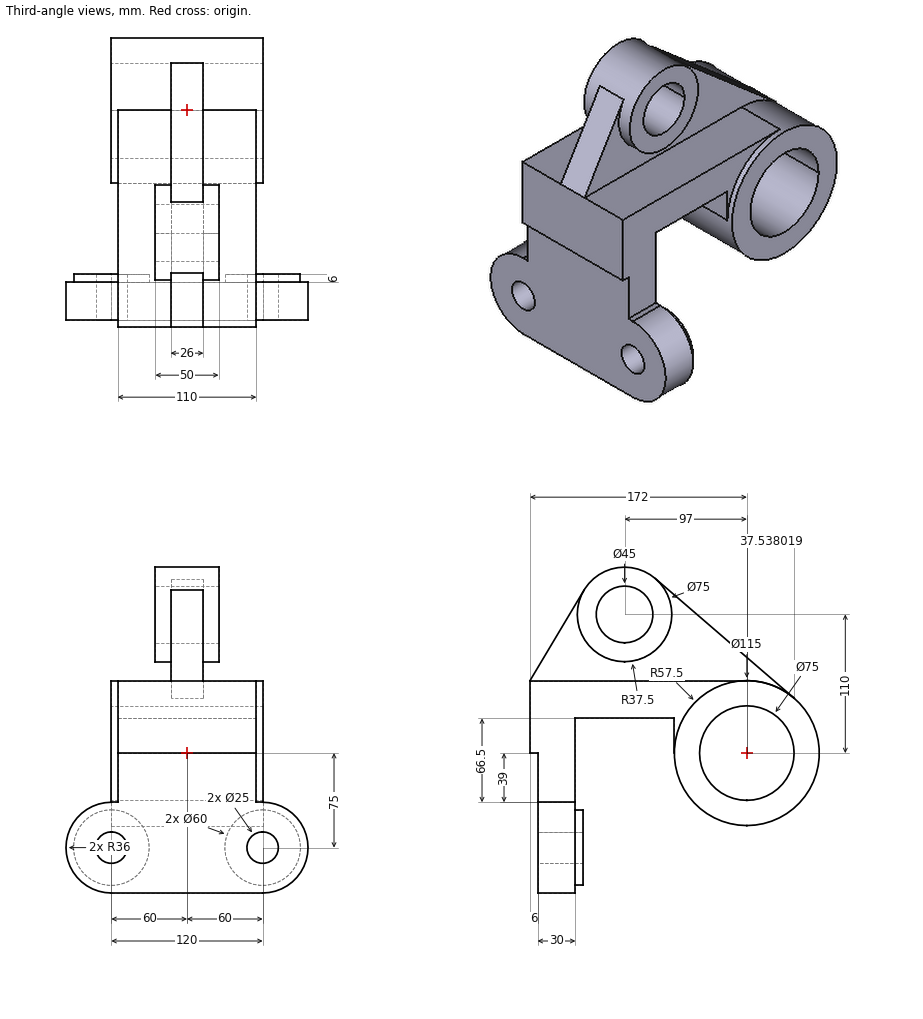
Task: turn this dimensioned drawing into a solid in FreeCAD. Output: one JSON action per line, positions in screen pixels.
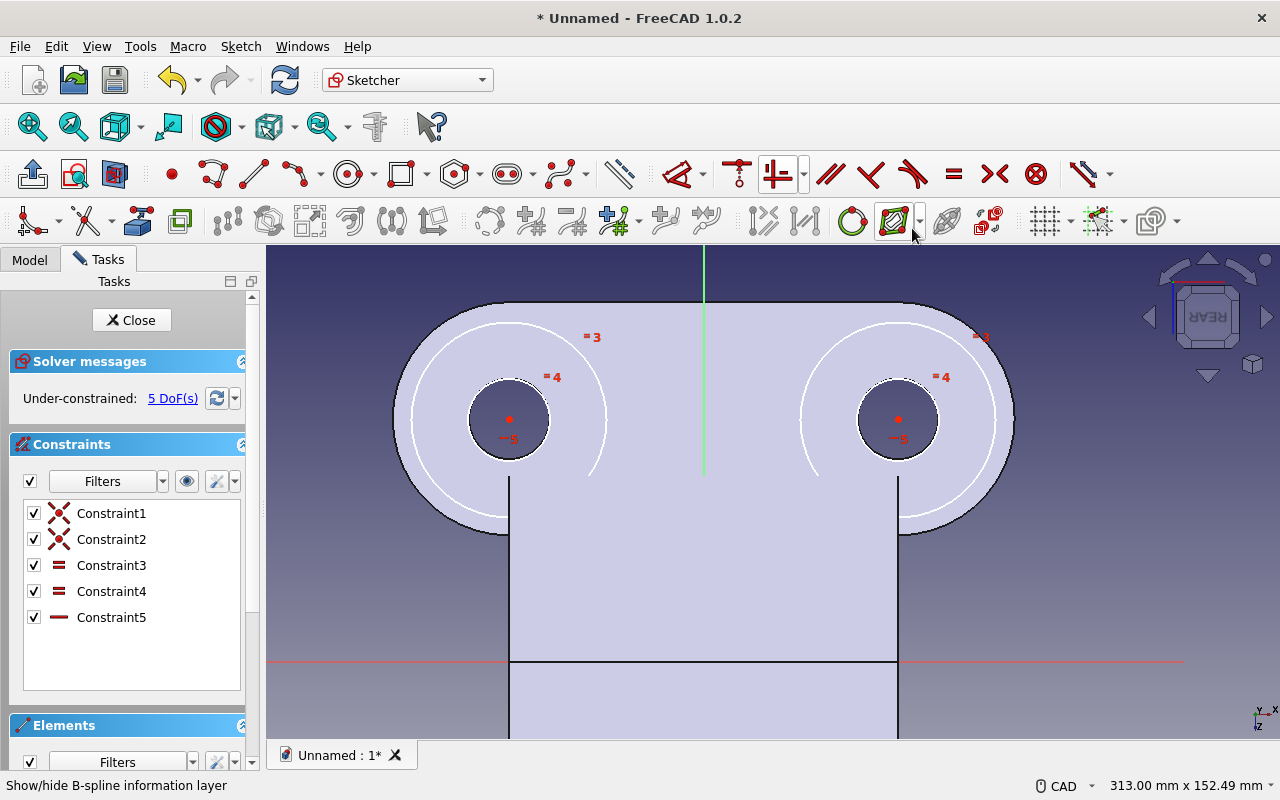
{"action": "left_click", "coordinate": [676, 174]}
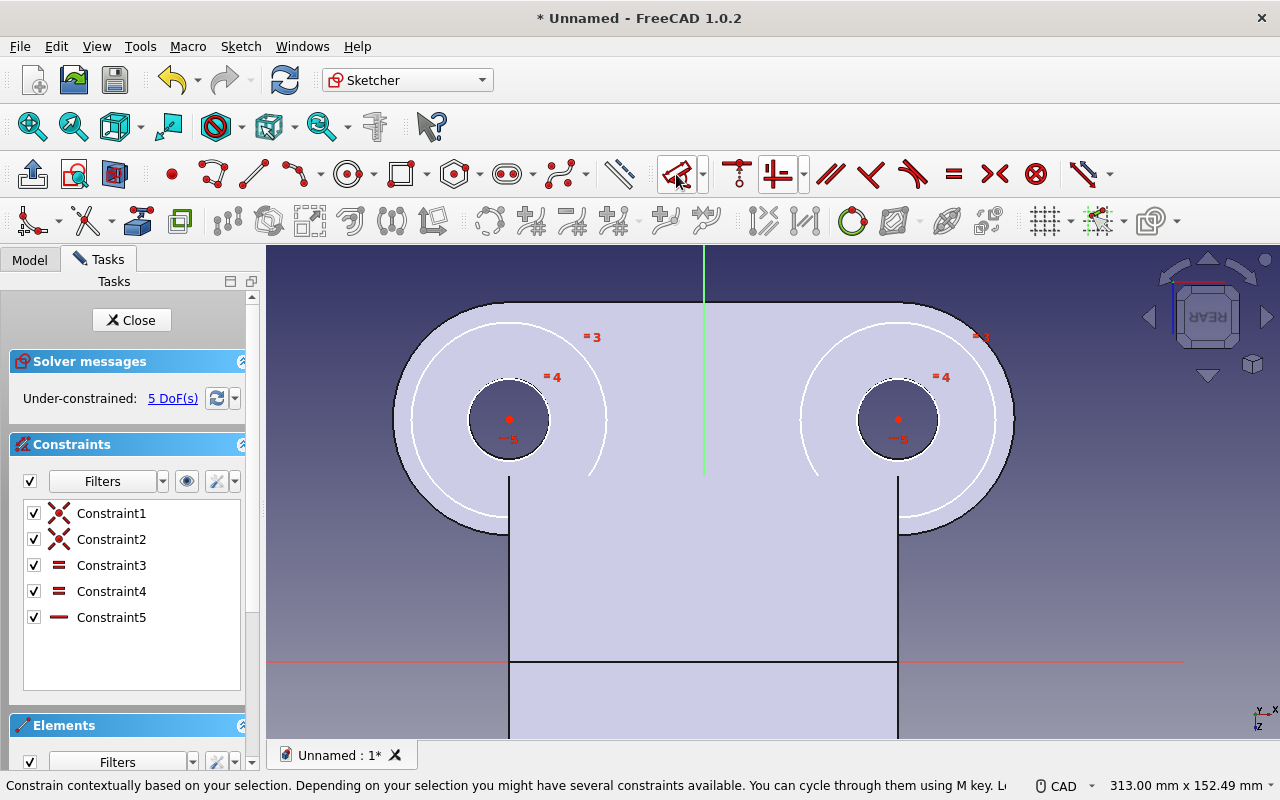
{"action": "left_click", "coordinate": [967, 351]}
{"action": "left_click", "coordinate": [990, 328]}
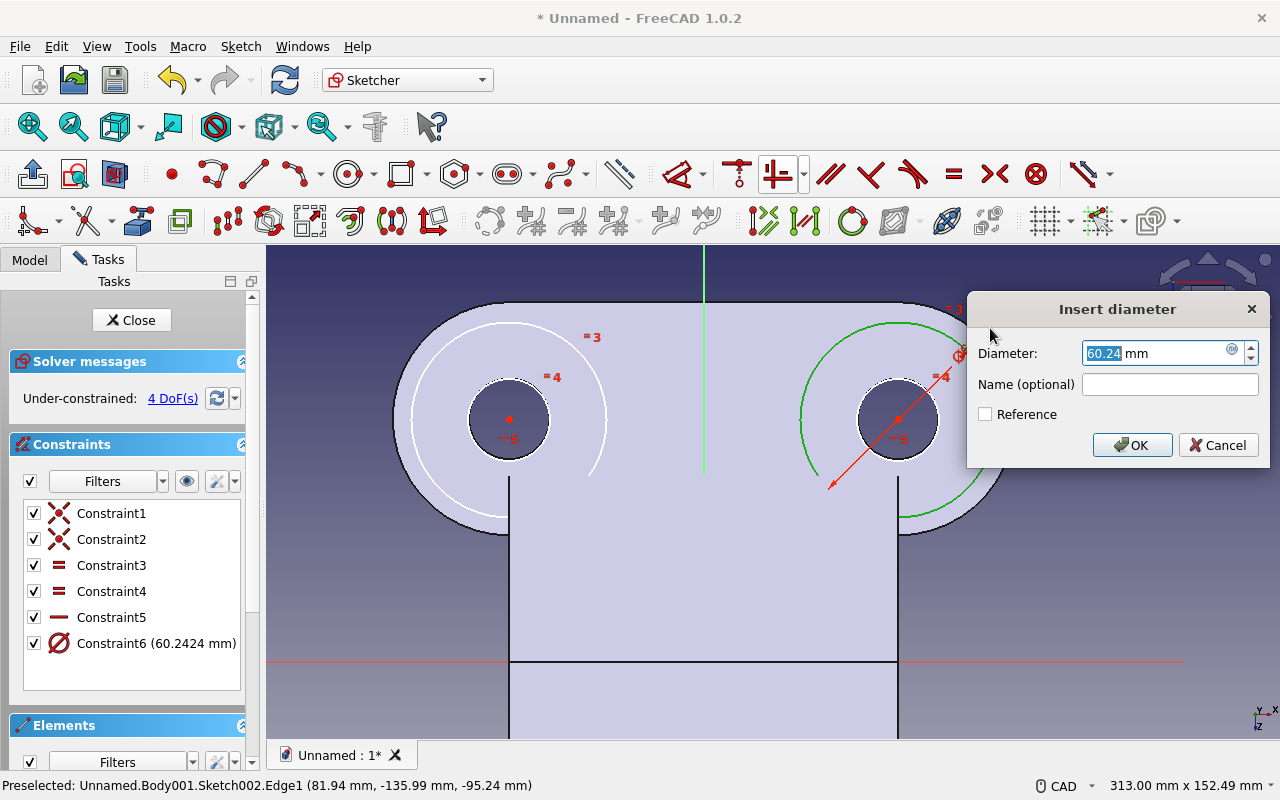
{"action": "type", "text": "60"}
{"action": "key", "text": "Return"}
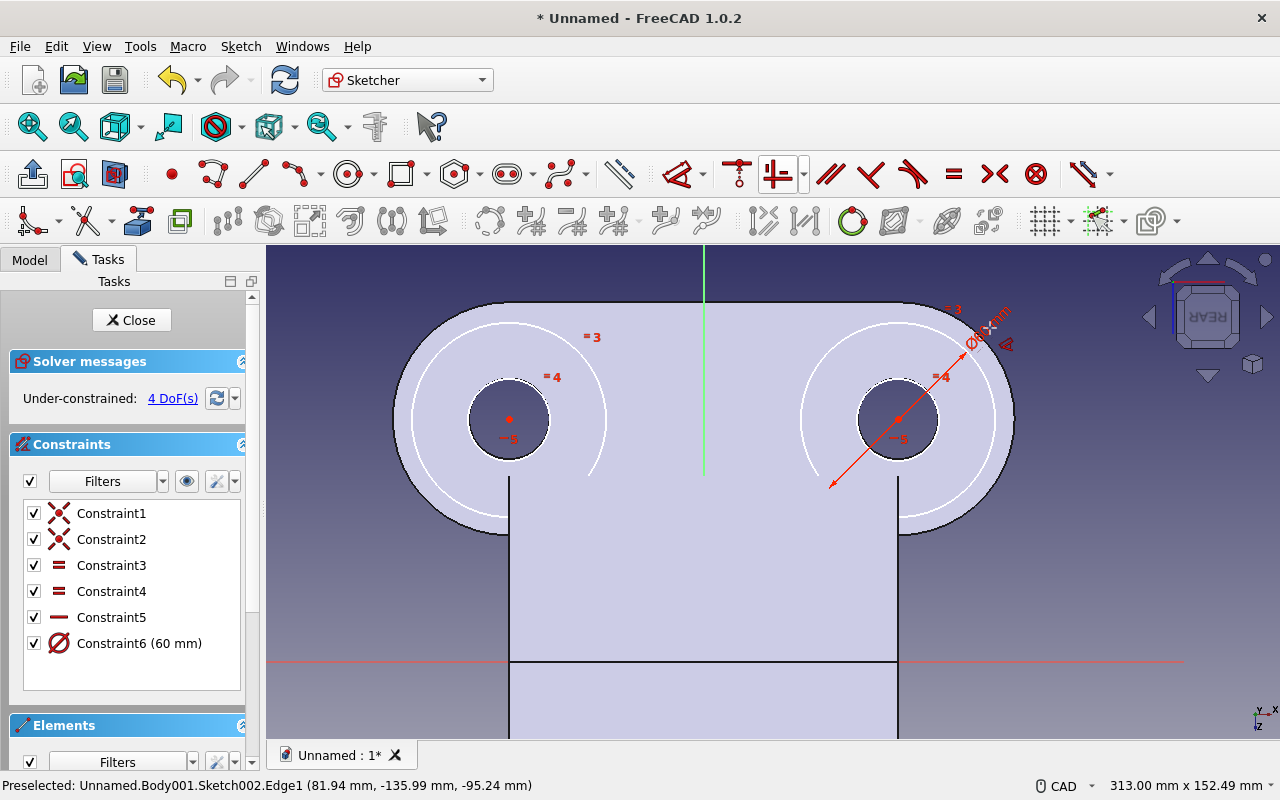
{"action": "left_click", "coordinate": [927, 391]}
{"action": "left_click", "coordinate": [950, 368]}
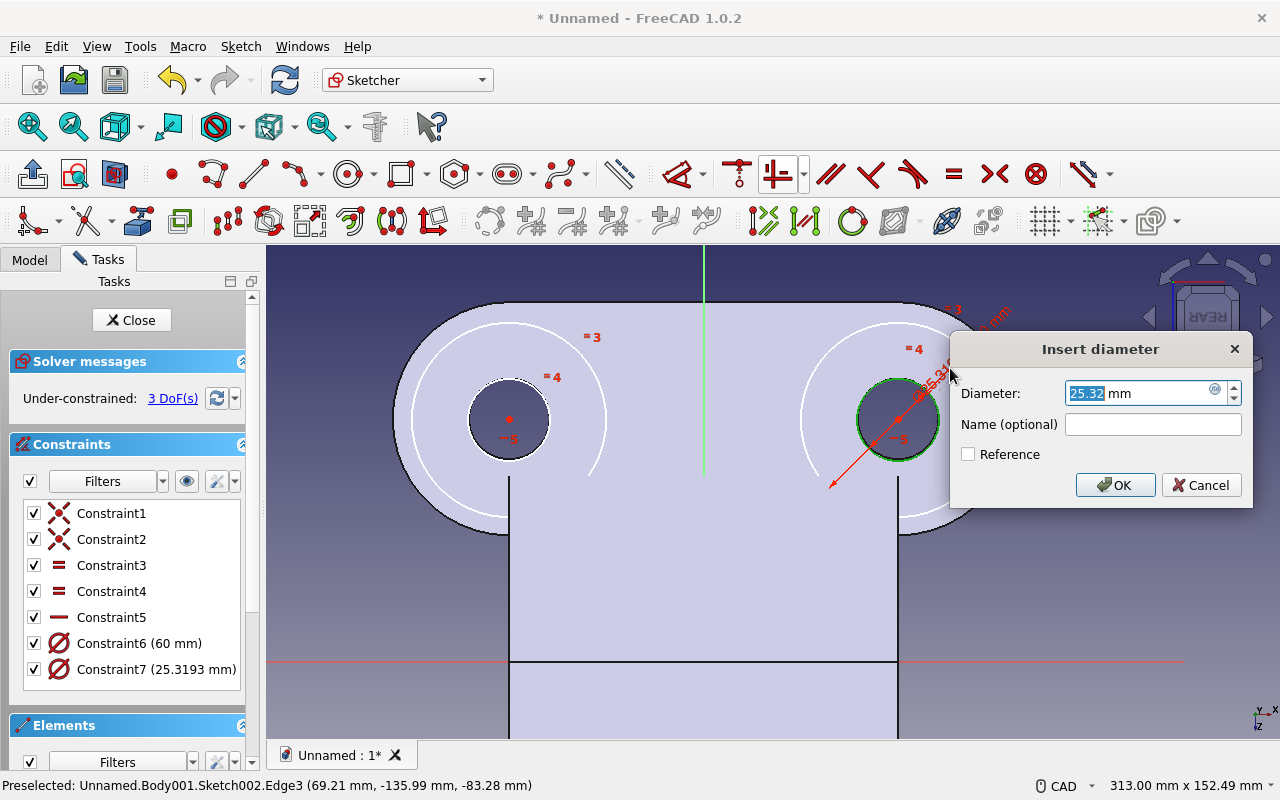
{"action": "type", "text": "25"}
{"action": "key", "text": "Return"}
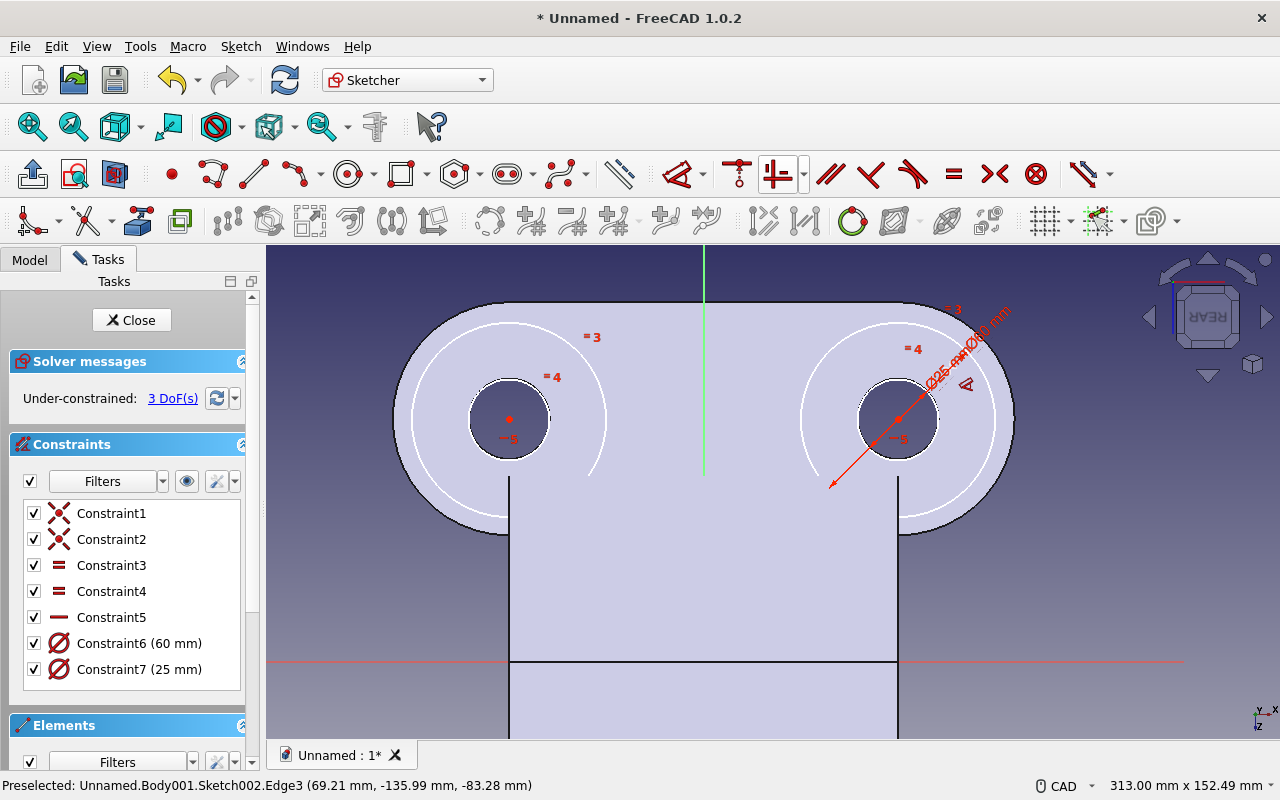
{"action": "left_click", "coordinate": [898, 420]}
{"action": "left_click", "coordinate": [801, 696]}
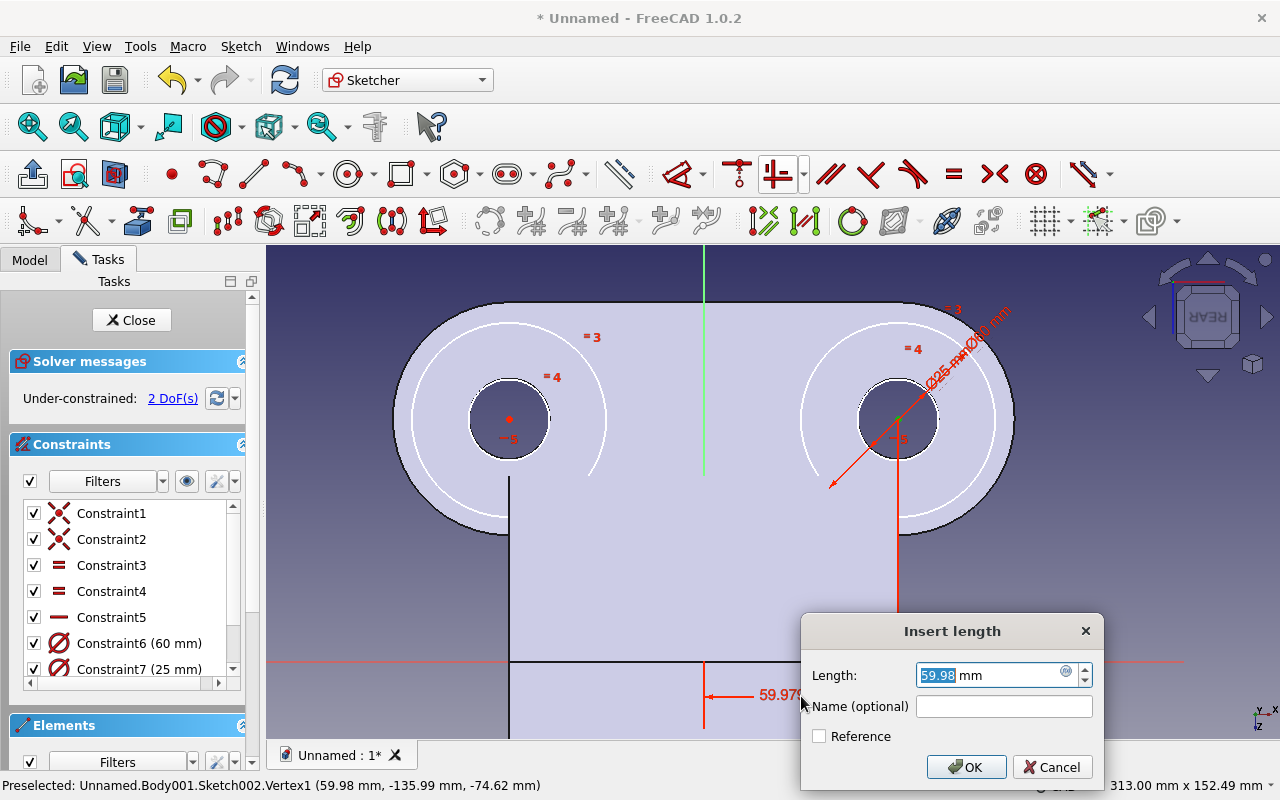
{"action": "type", "text": "60"}
{"action": "key", "text": "Return"}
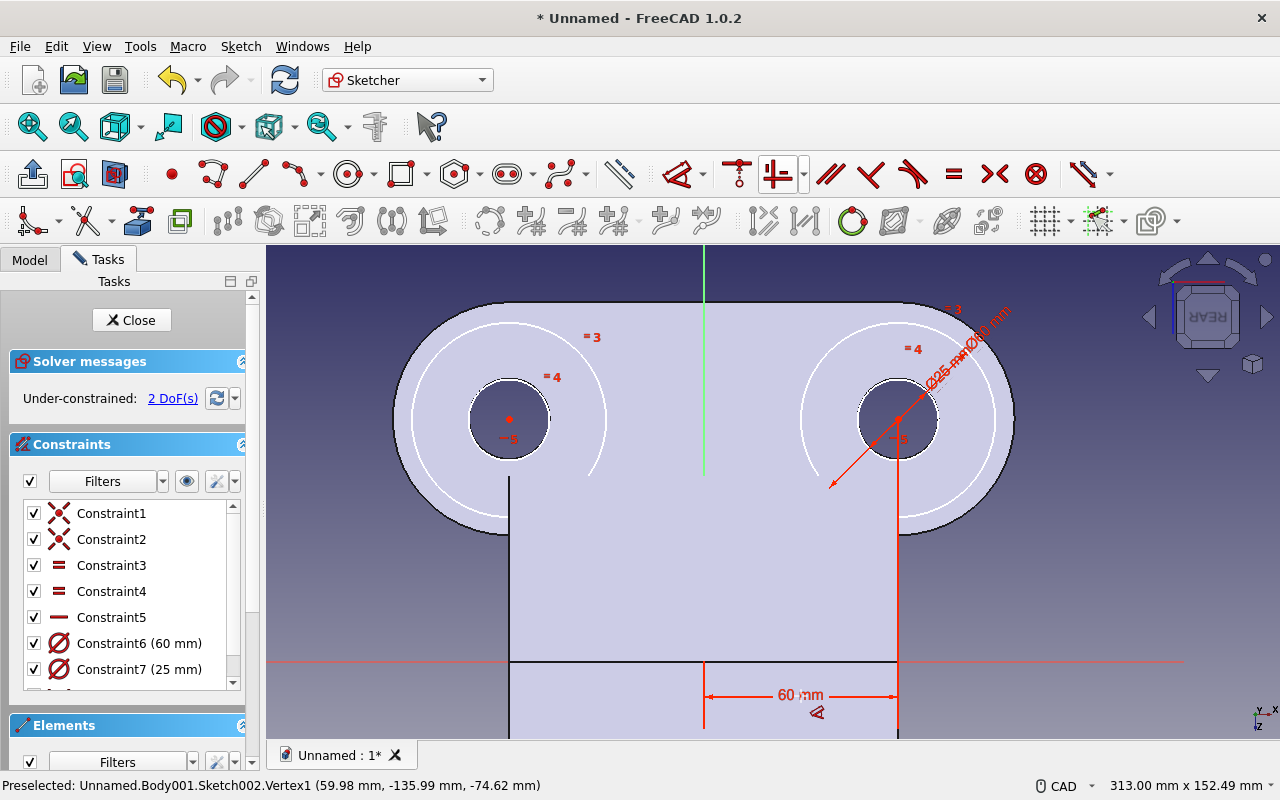
{"action": "left_click", "coordinate": [898, 420]}
{"action": "left_click", "coordinate": [932, 541]}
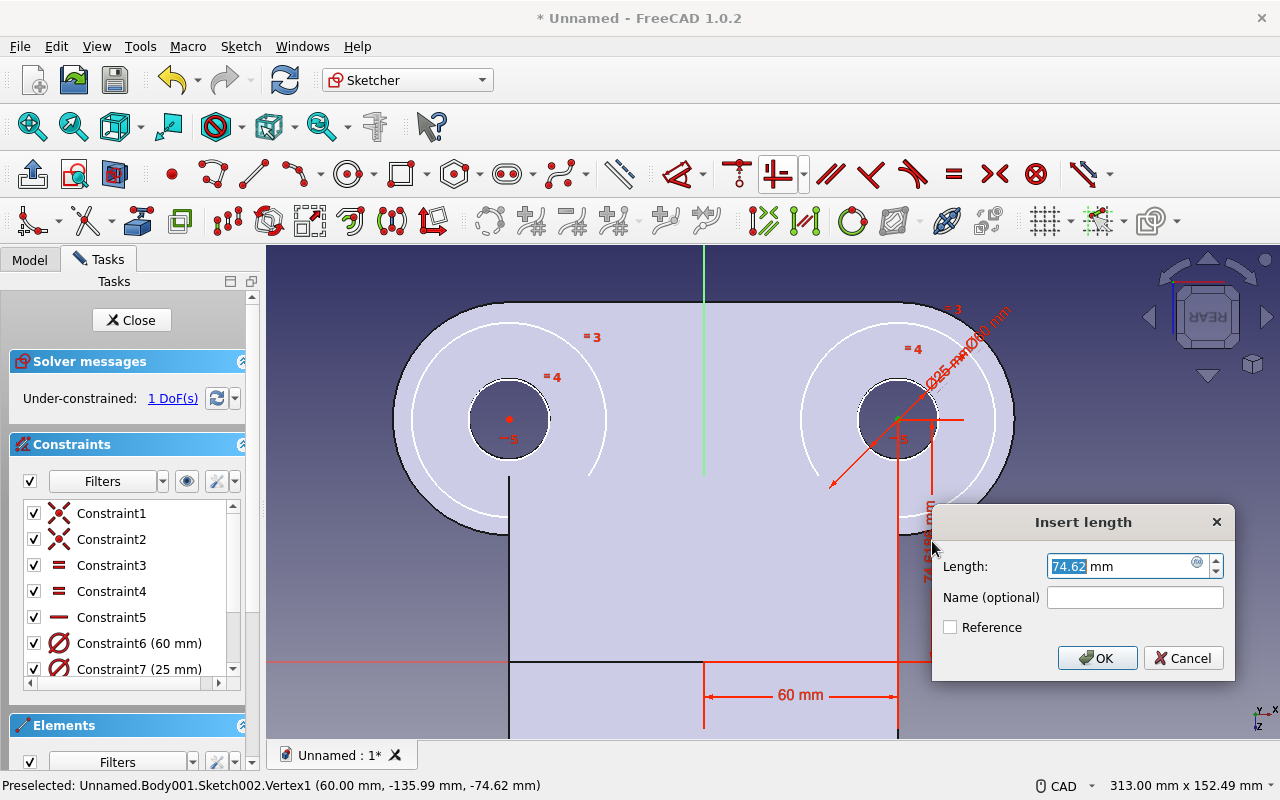
{"action": "type", "text": "75"}
{"action": "key", "text": "Return"}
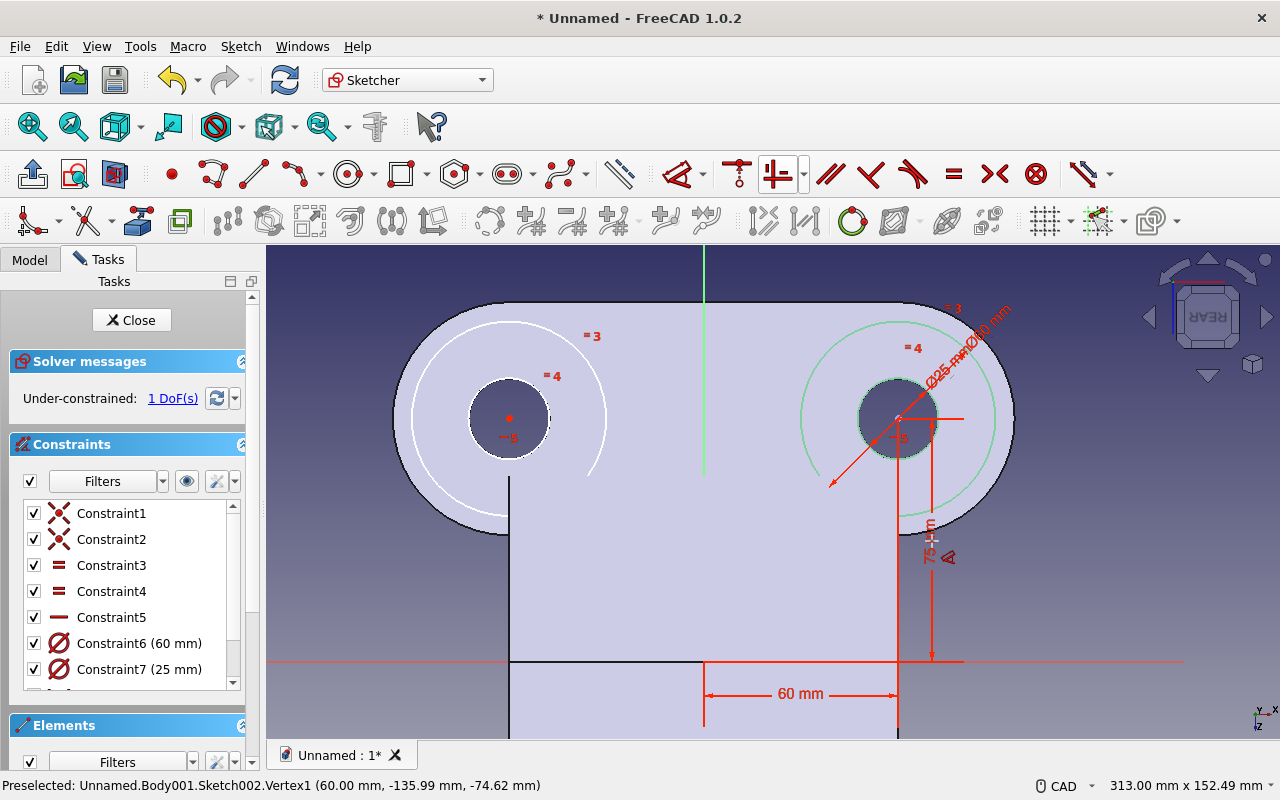
{"action": "left_click", "coordinate": [509, 419]}
{"action": "left_click", "coordinate": [606, 696]}